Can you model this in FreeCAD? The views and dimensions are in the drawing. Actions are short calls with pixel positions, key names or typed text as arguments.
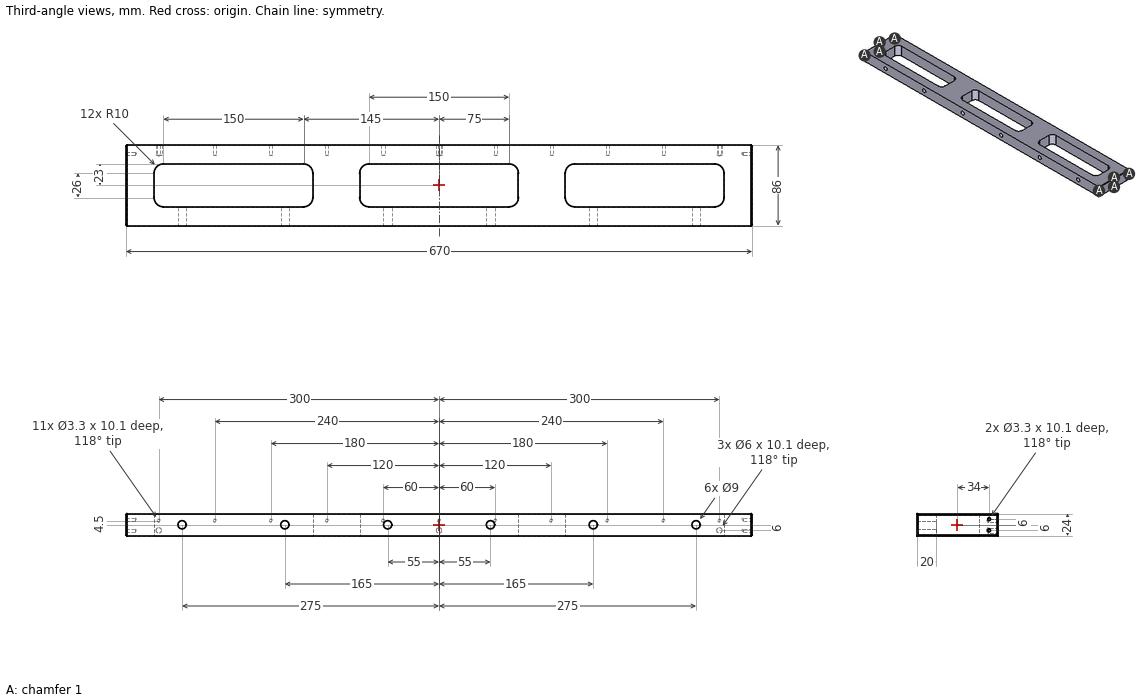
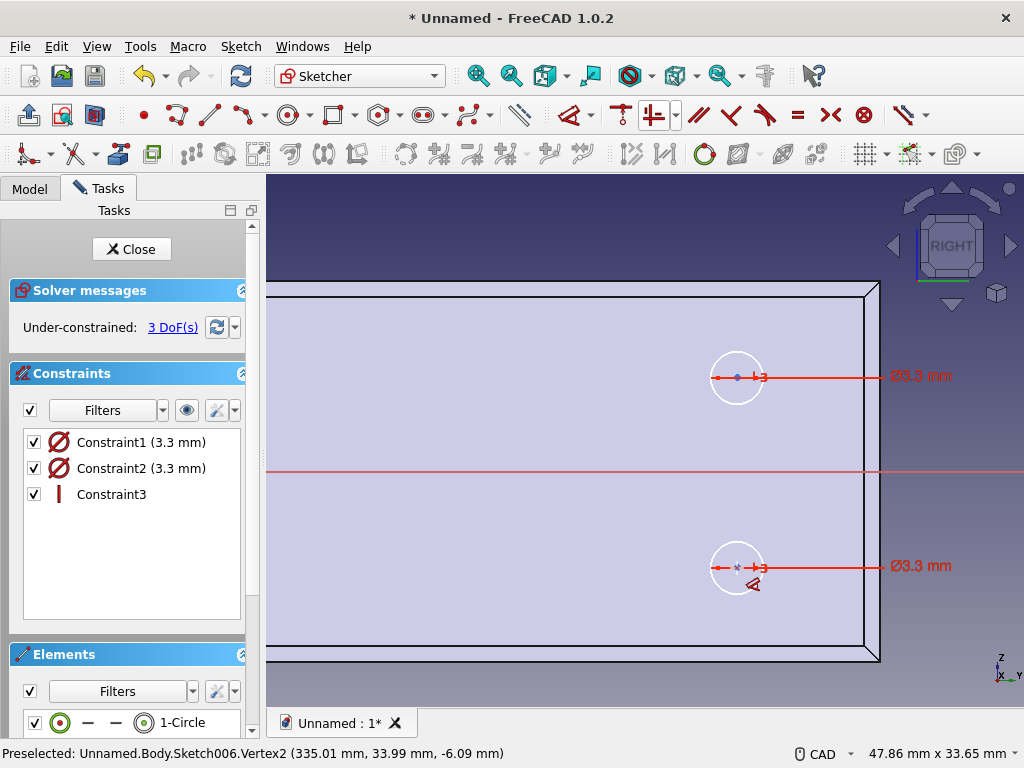
click(737, 378)
click(771, 425)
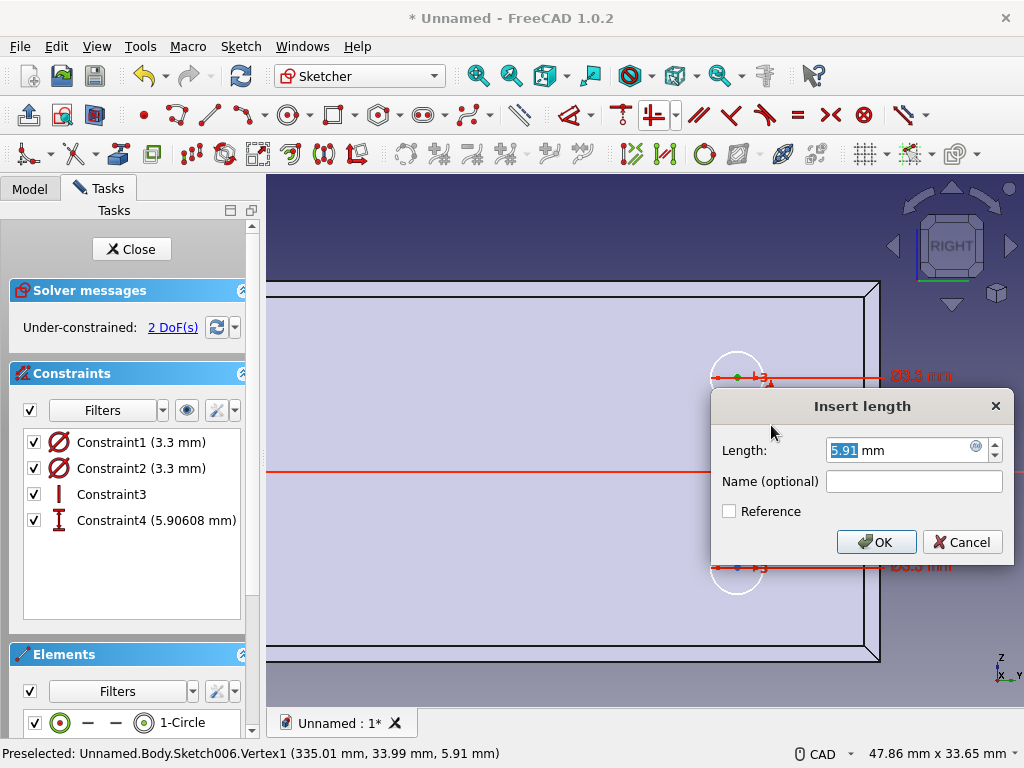
text(6)
key(Return)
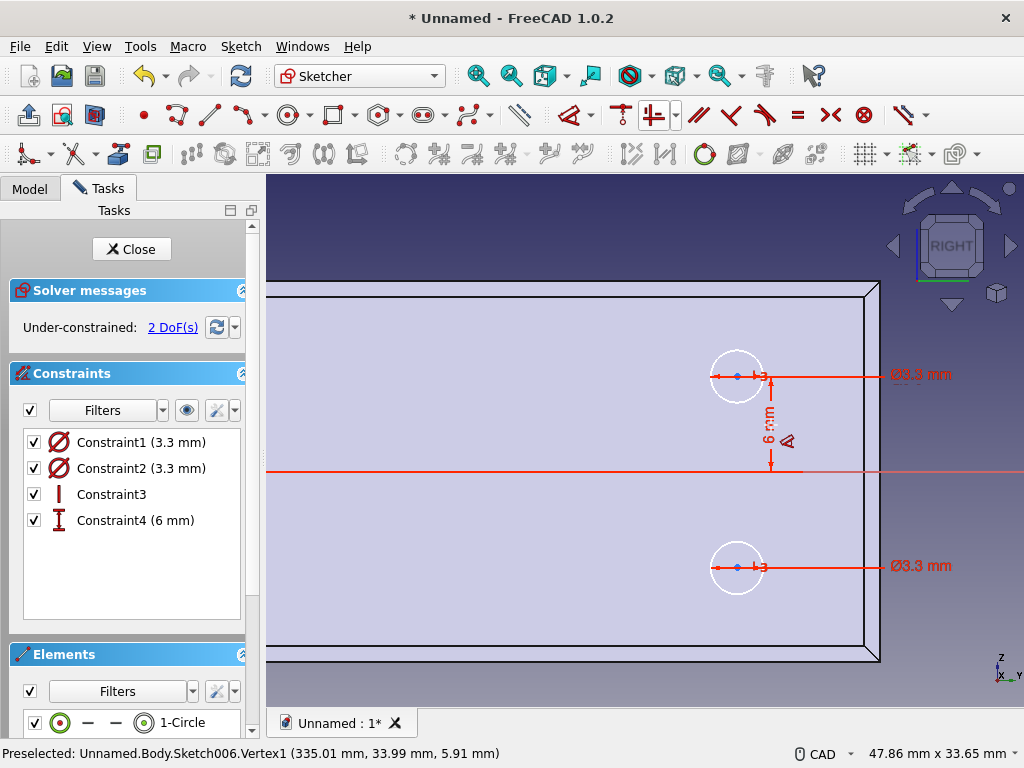
click(737, 568)
click(771, 520)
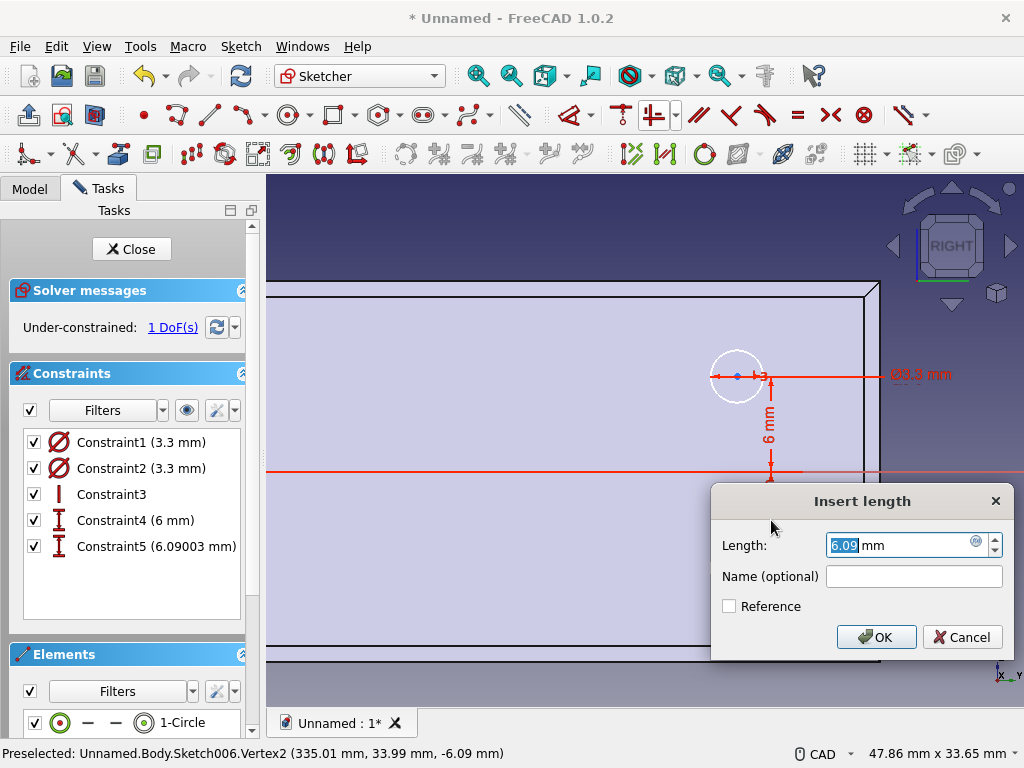
text(6)
key(Return)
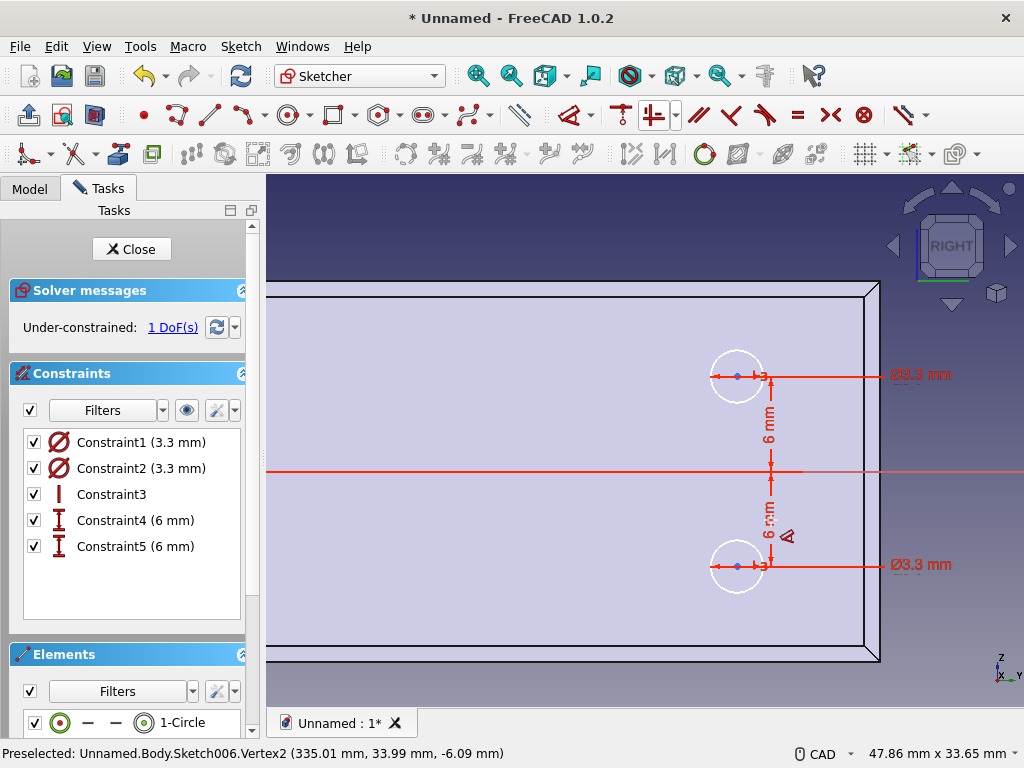
click(737, 377)
click(516, 343)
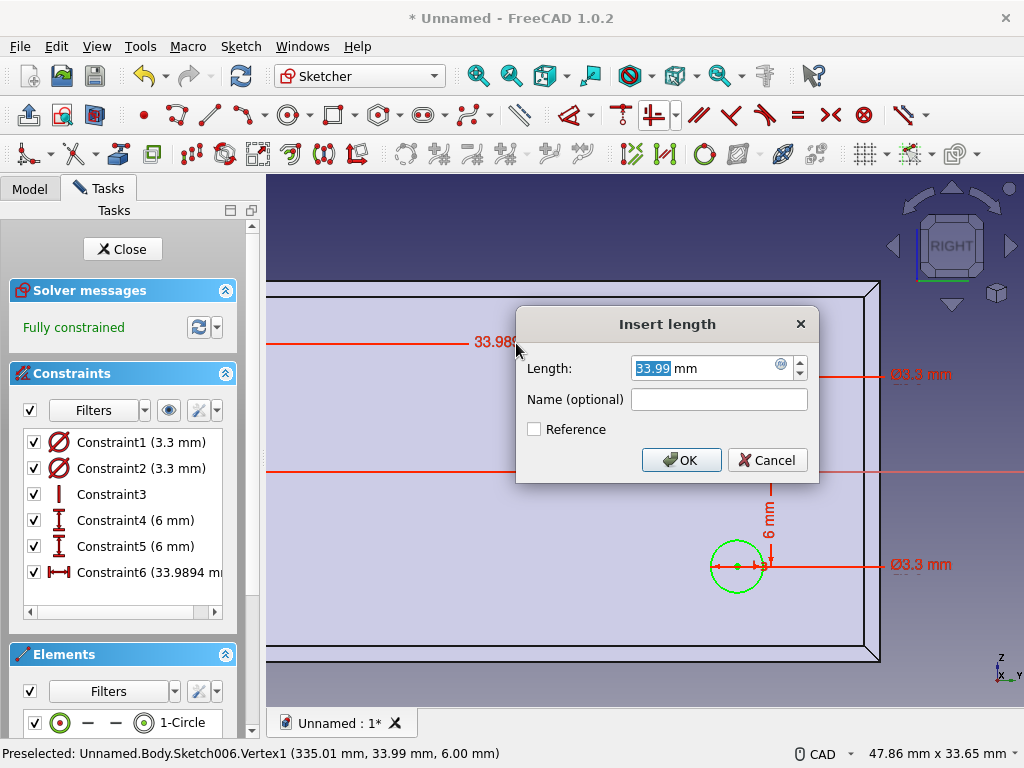
text(34)
key(Return)
key(Escape)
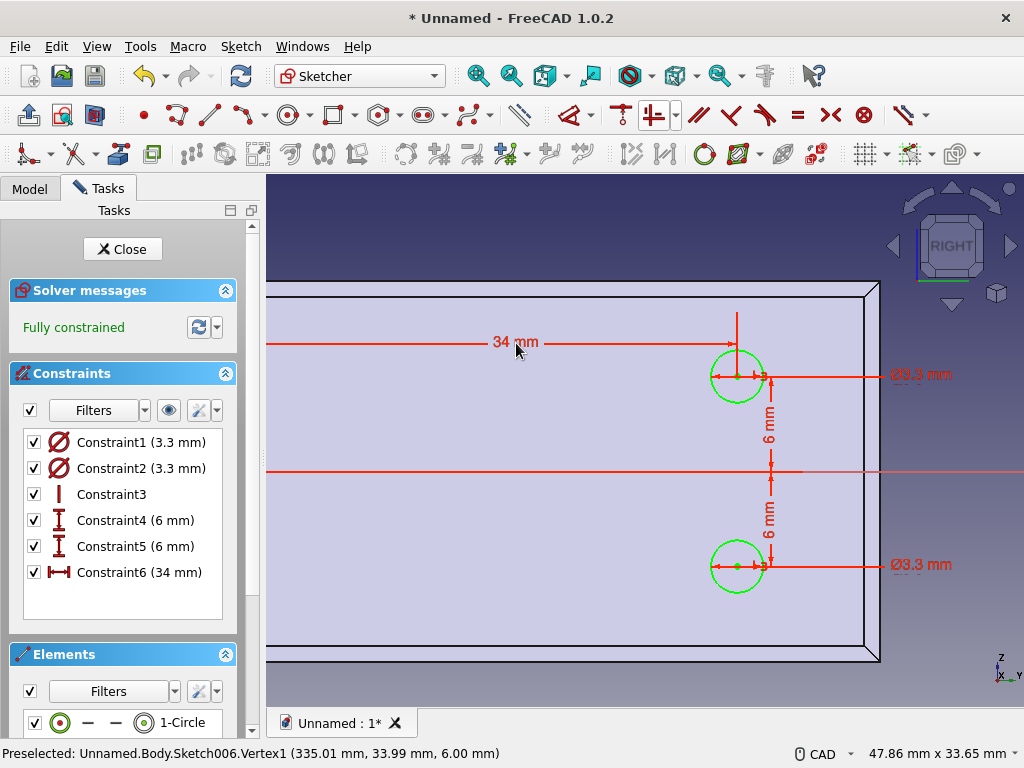
click(123, 249)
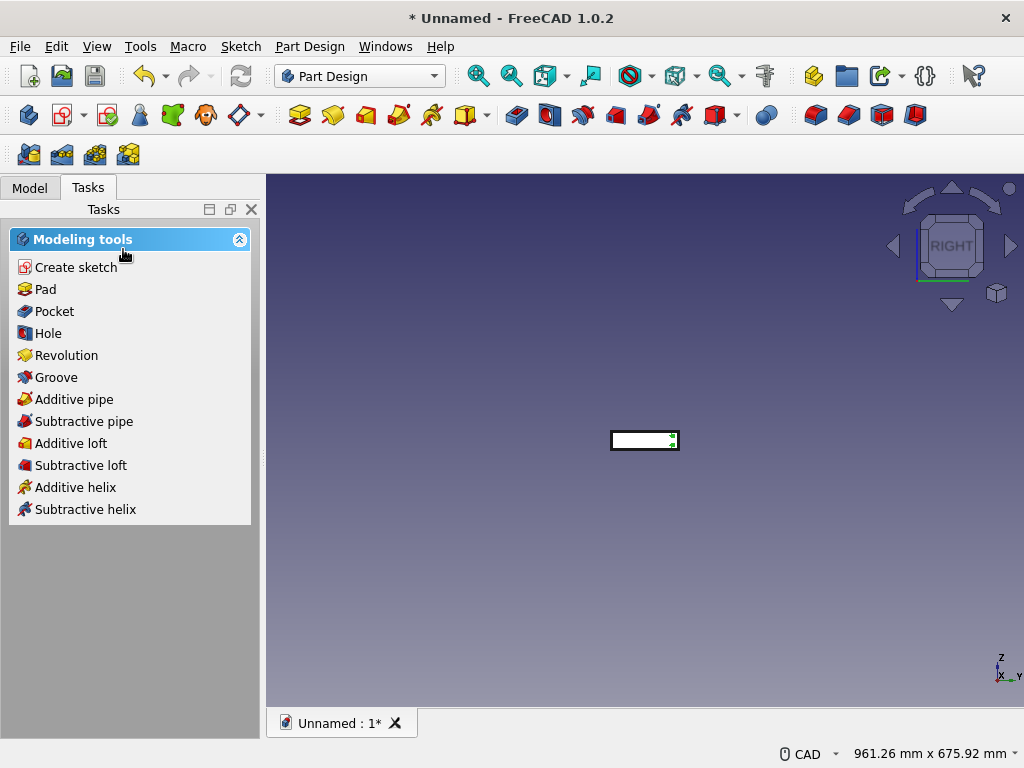
click(550, 116)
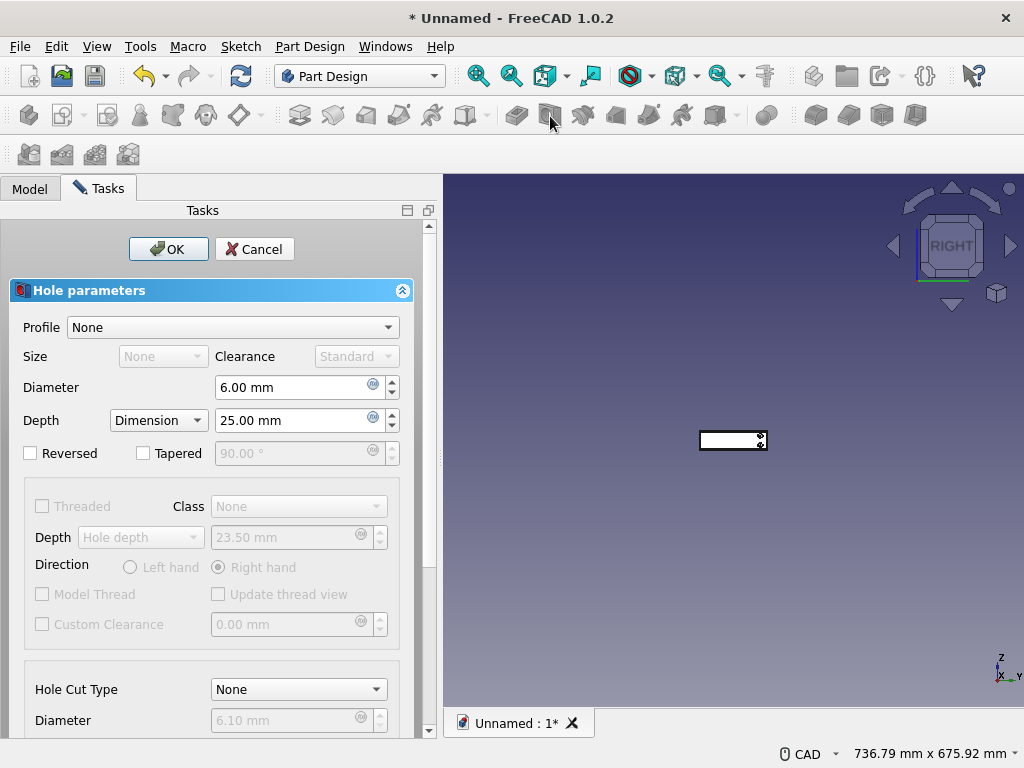
triple_click(300, 388)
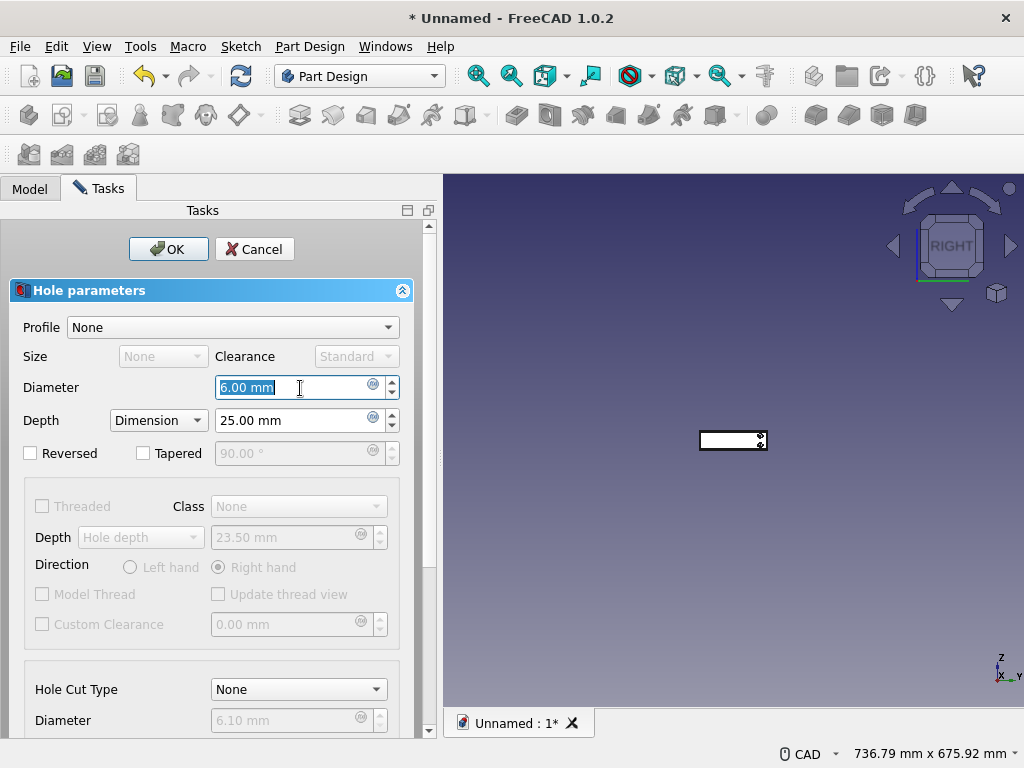
text(3.3)
key(Tab)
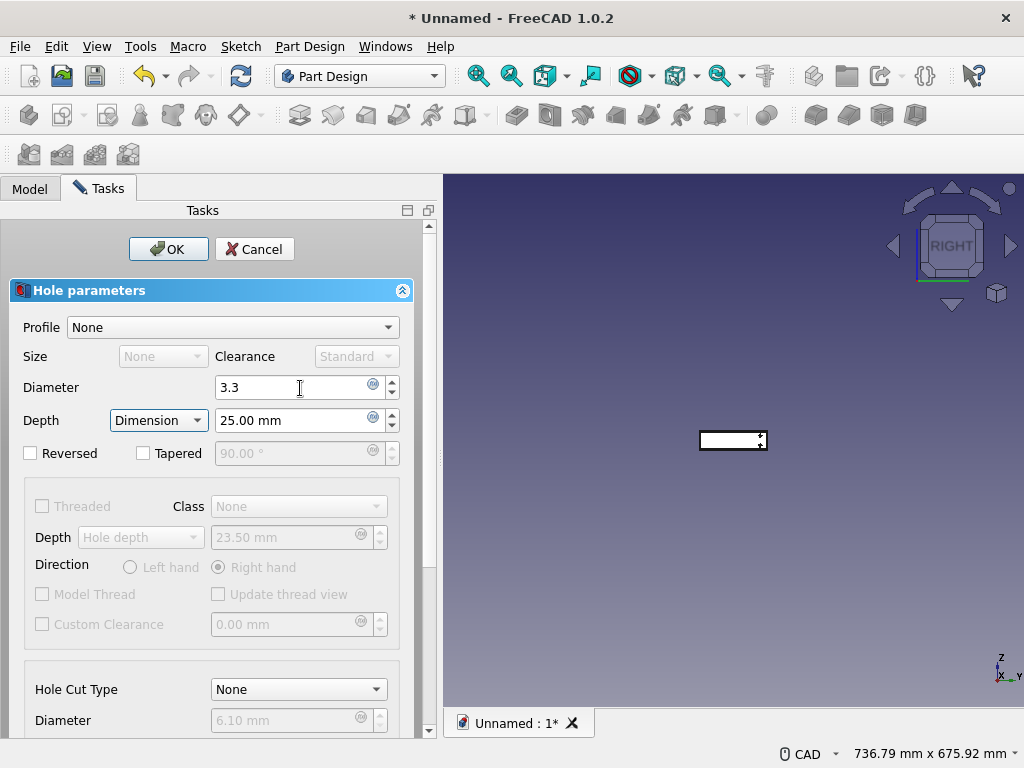
triple_click(300, 420)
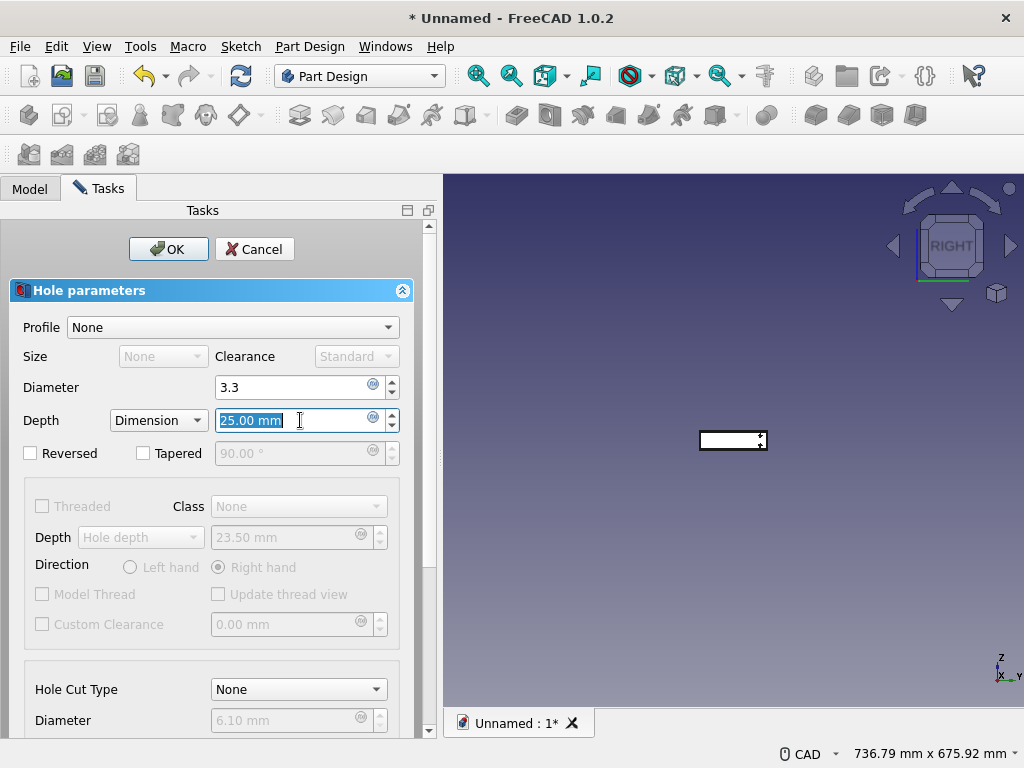
text(10.1)
key(Tab)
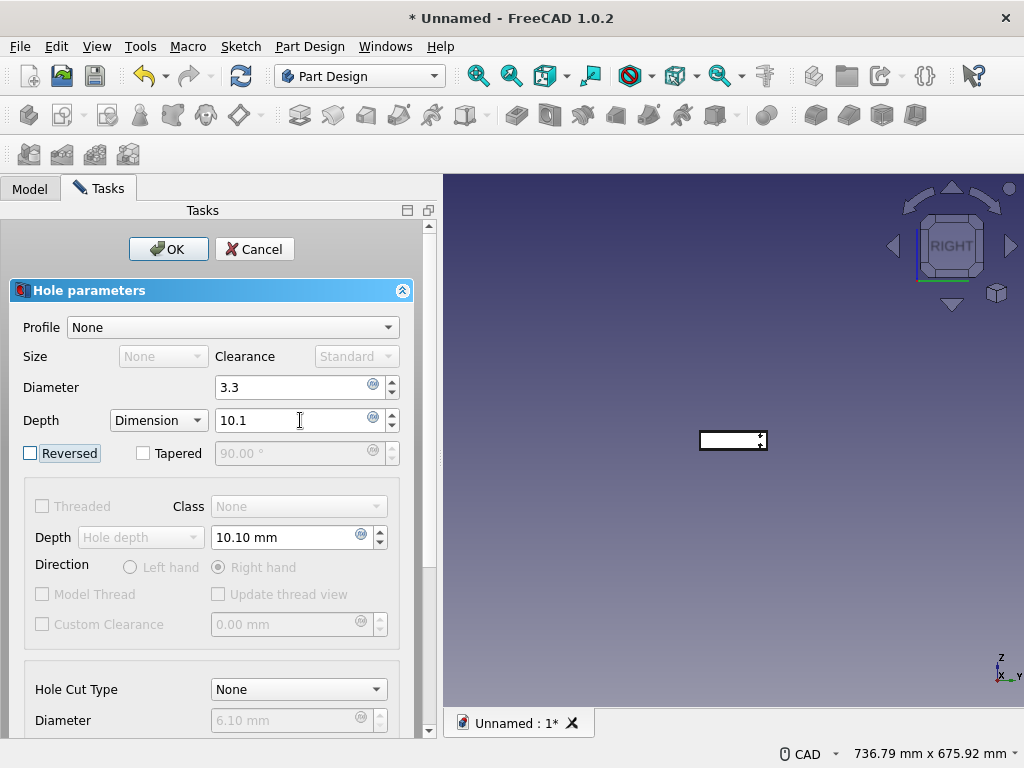
click(169, 249)